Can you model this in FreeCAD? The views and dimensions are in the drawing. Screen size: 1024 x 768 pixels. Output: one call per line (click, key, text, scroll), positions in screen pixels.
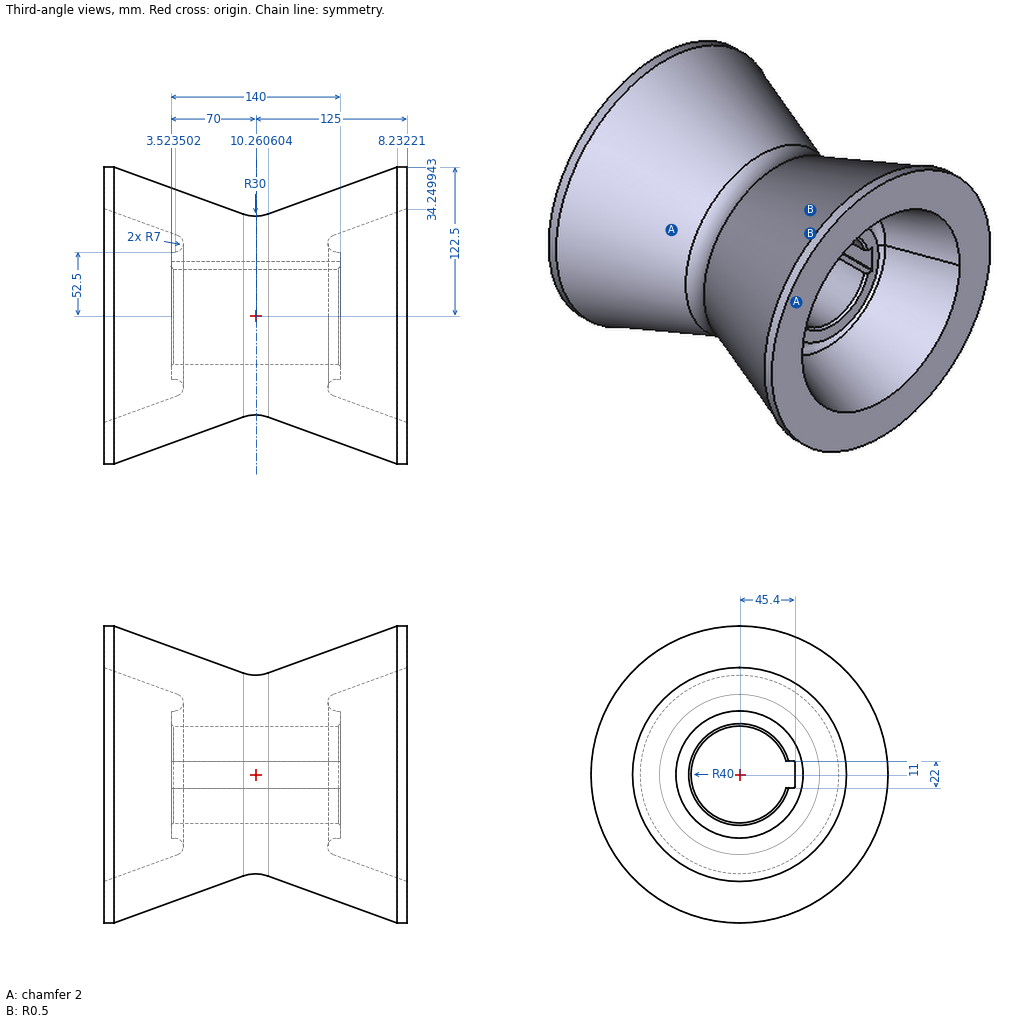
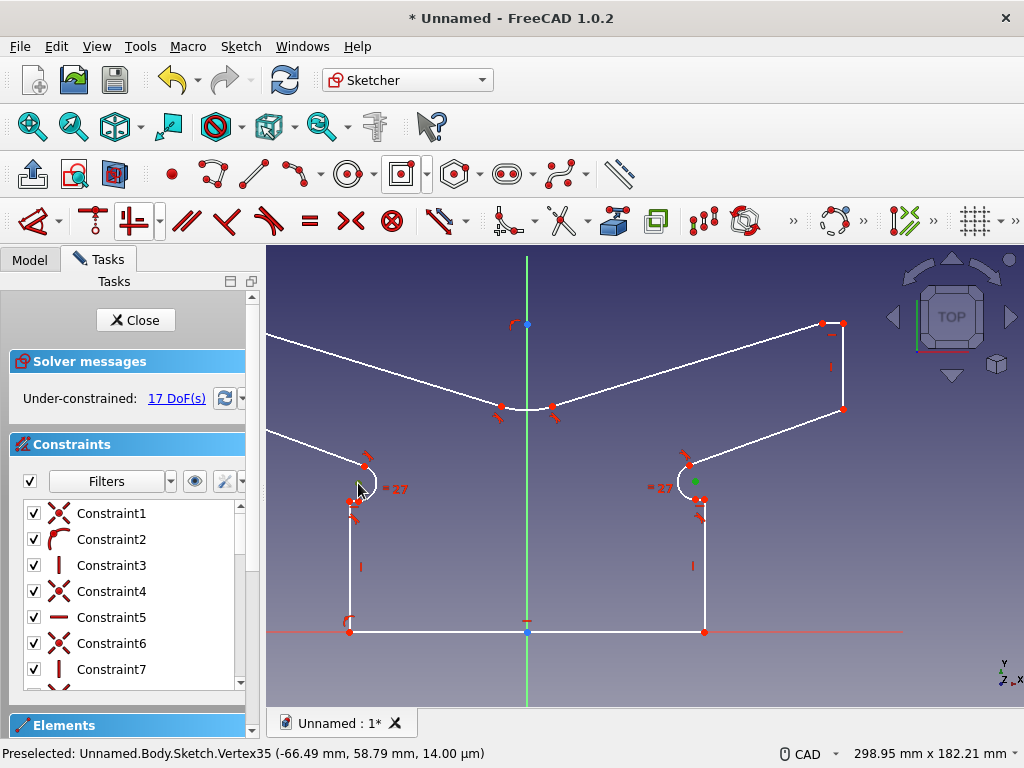
click(527, 592)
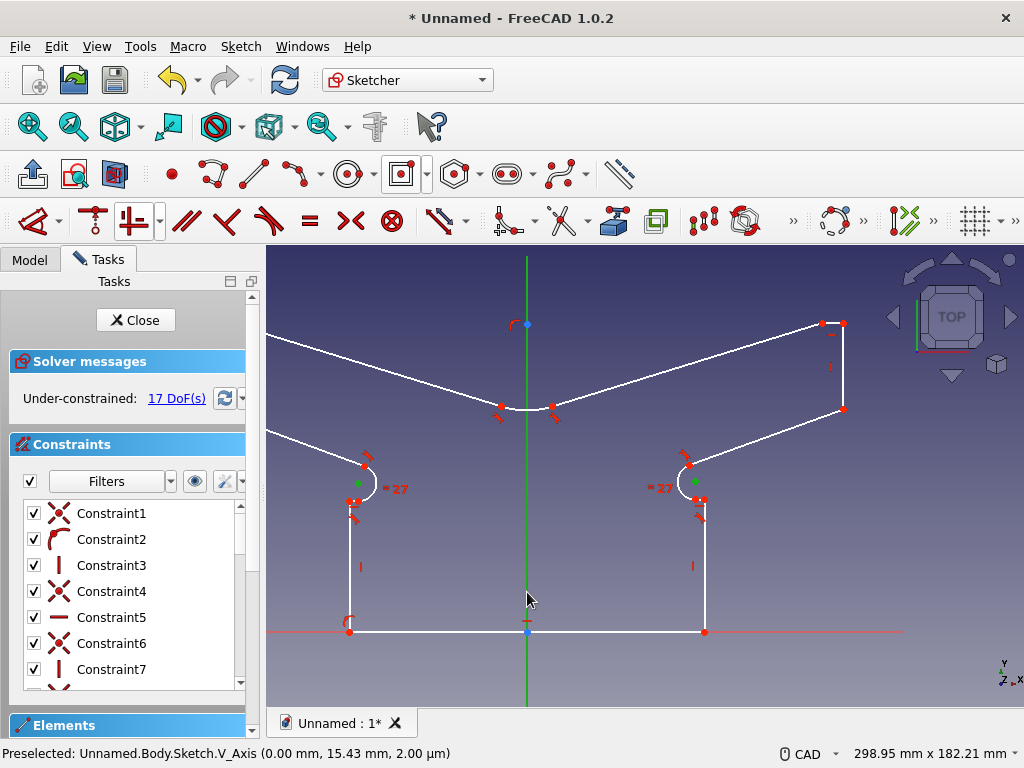
key(s)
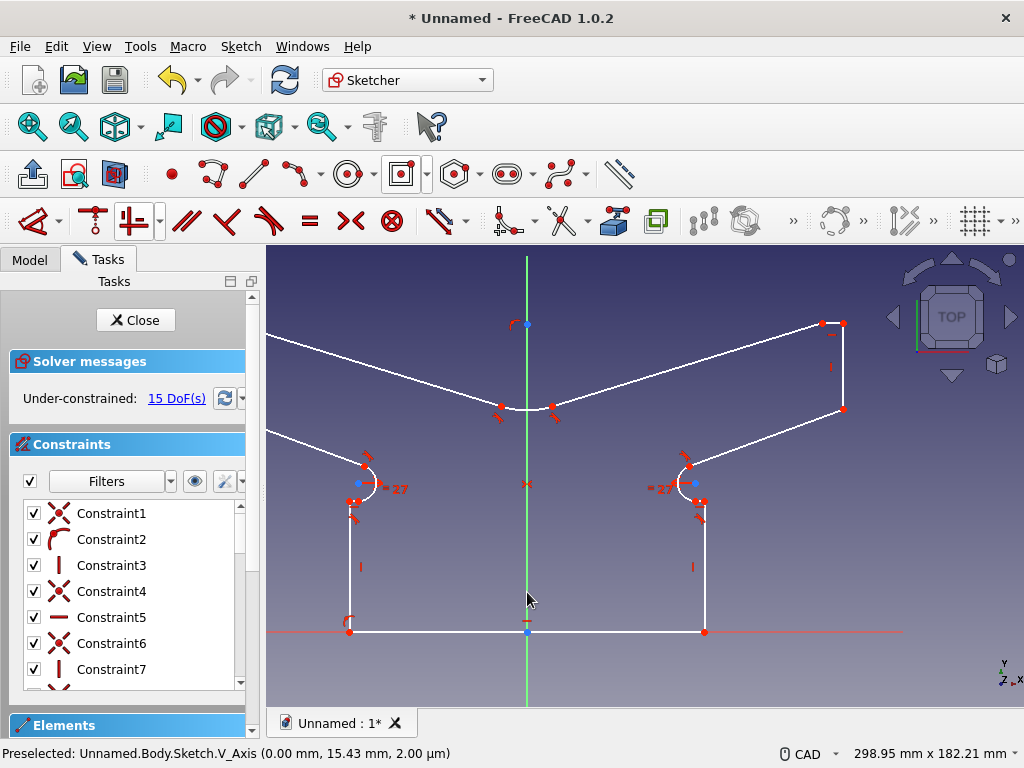
click(822, 323)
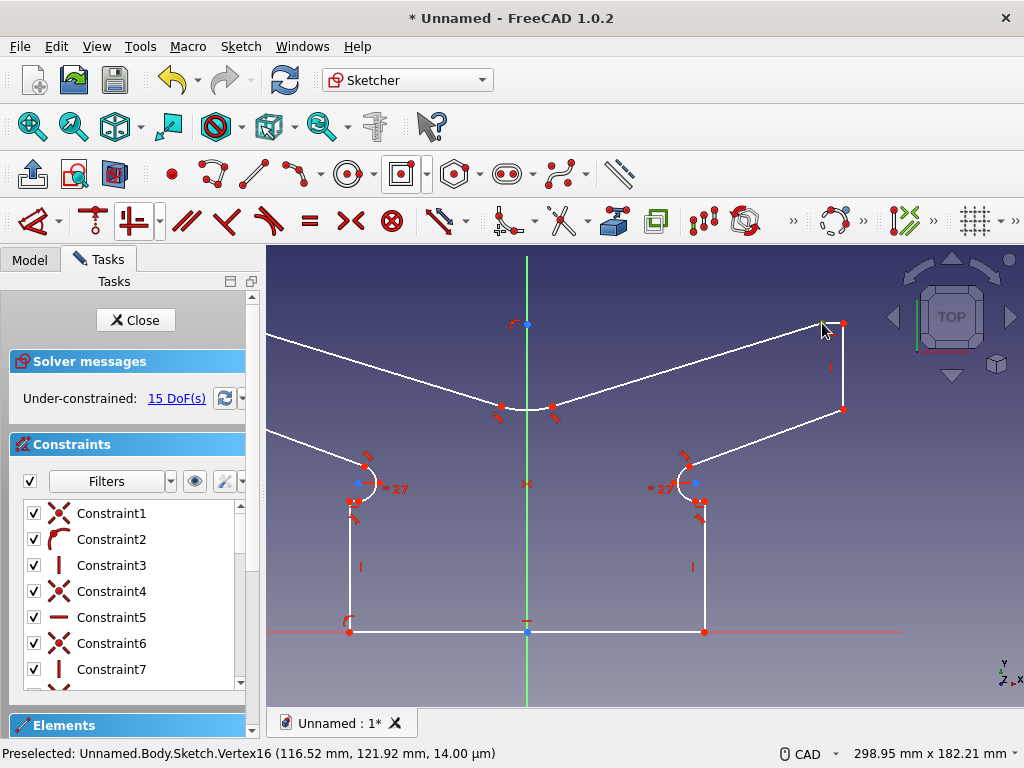
scroll(677, 474, down, 2)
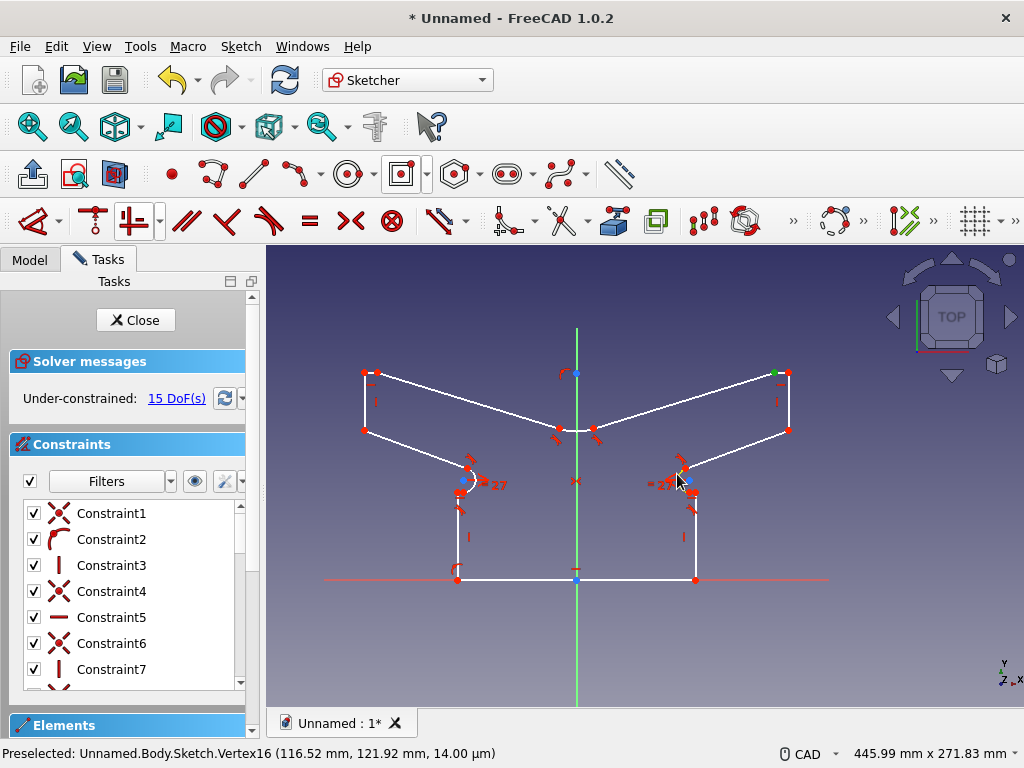
click(378, 373)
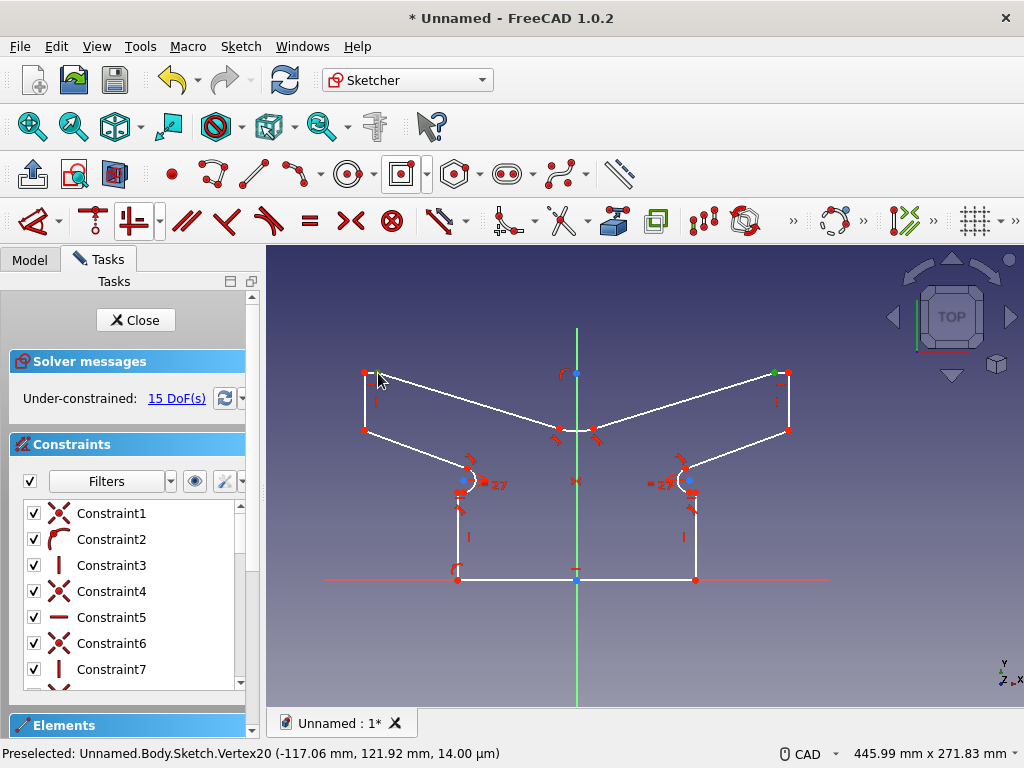
click(577, 650)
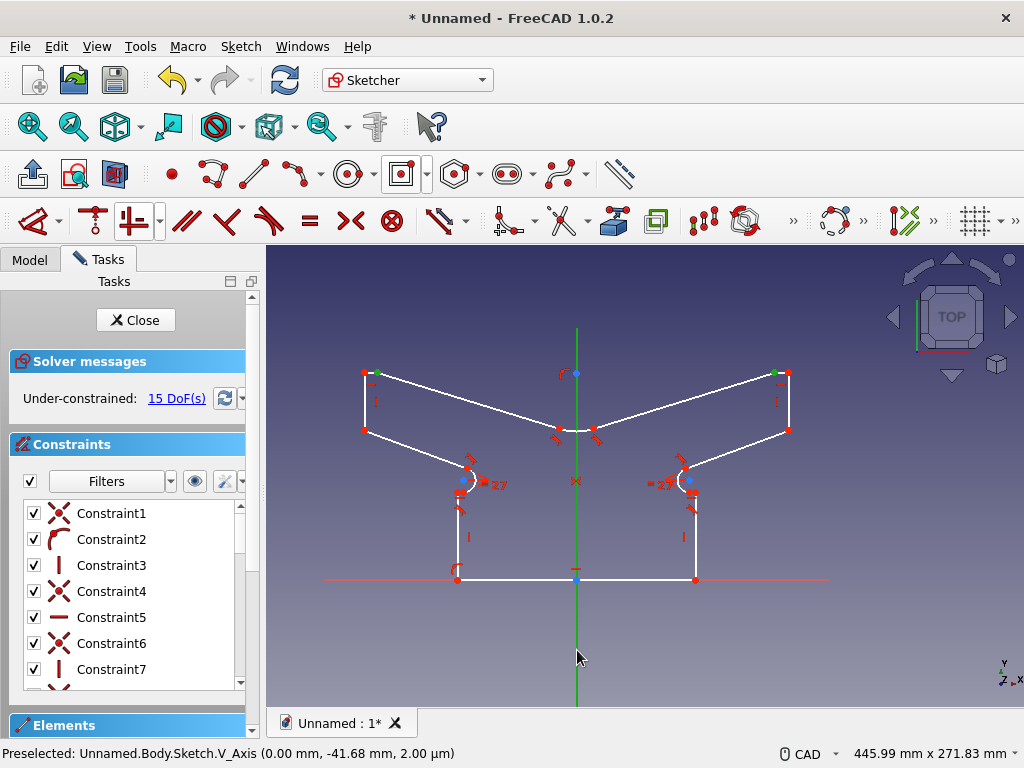
click(351, 222)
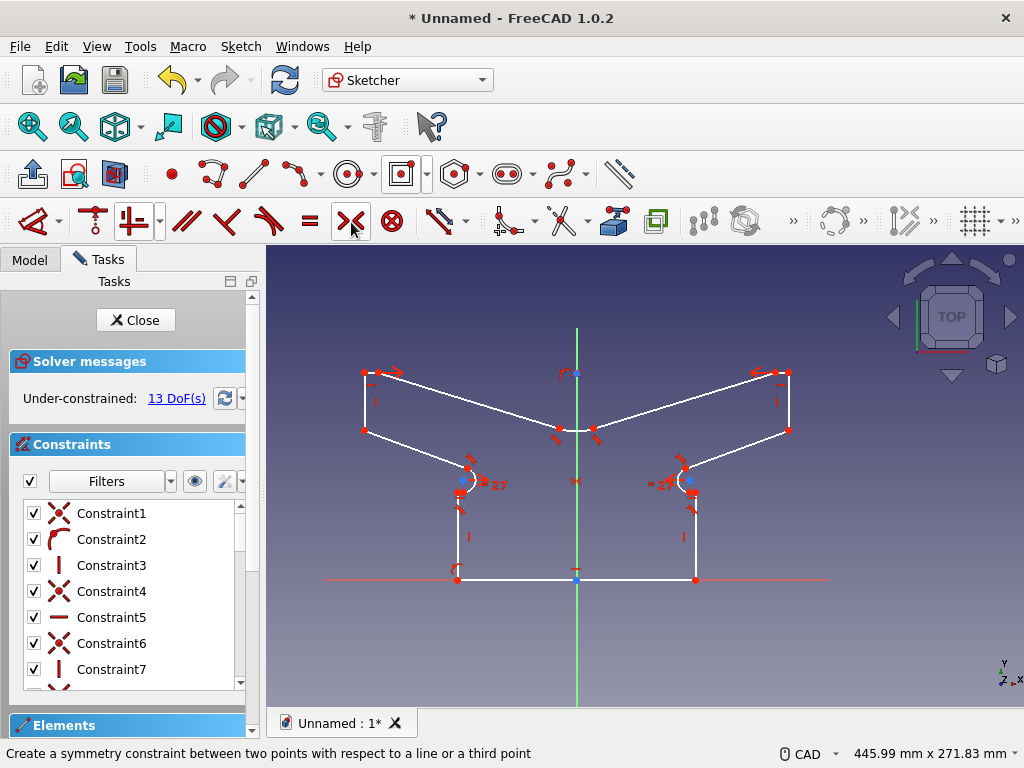
click(789, 431)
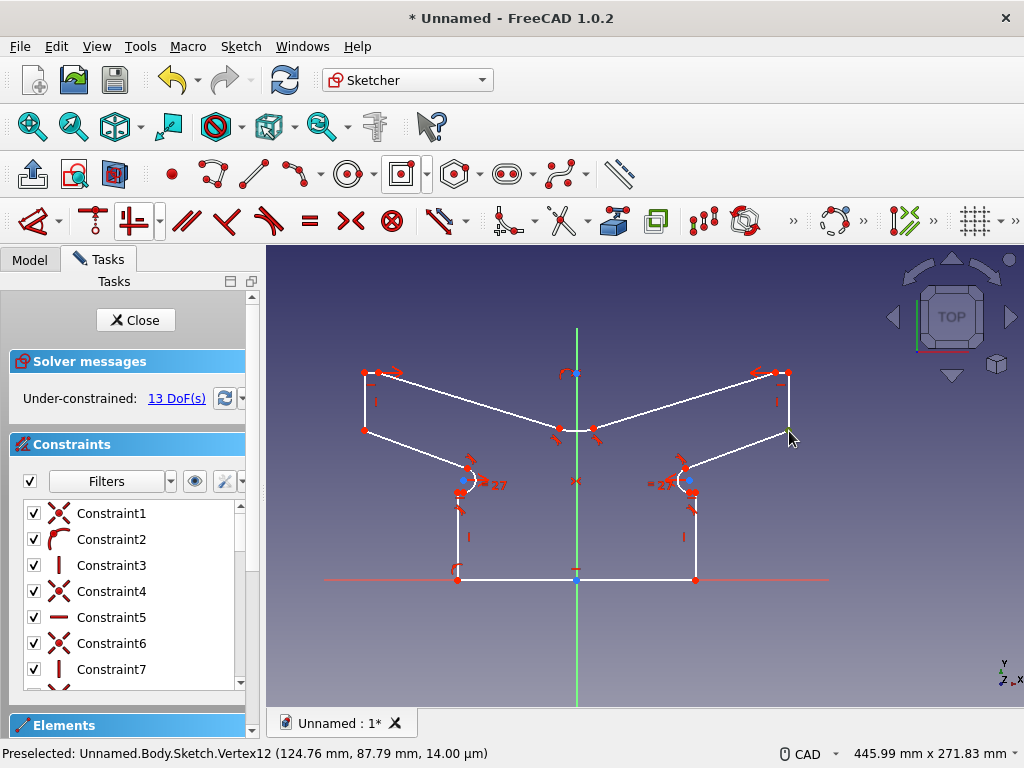
click(365, 431)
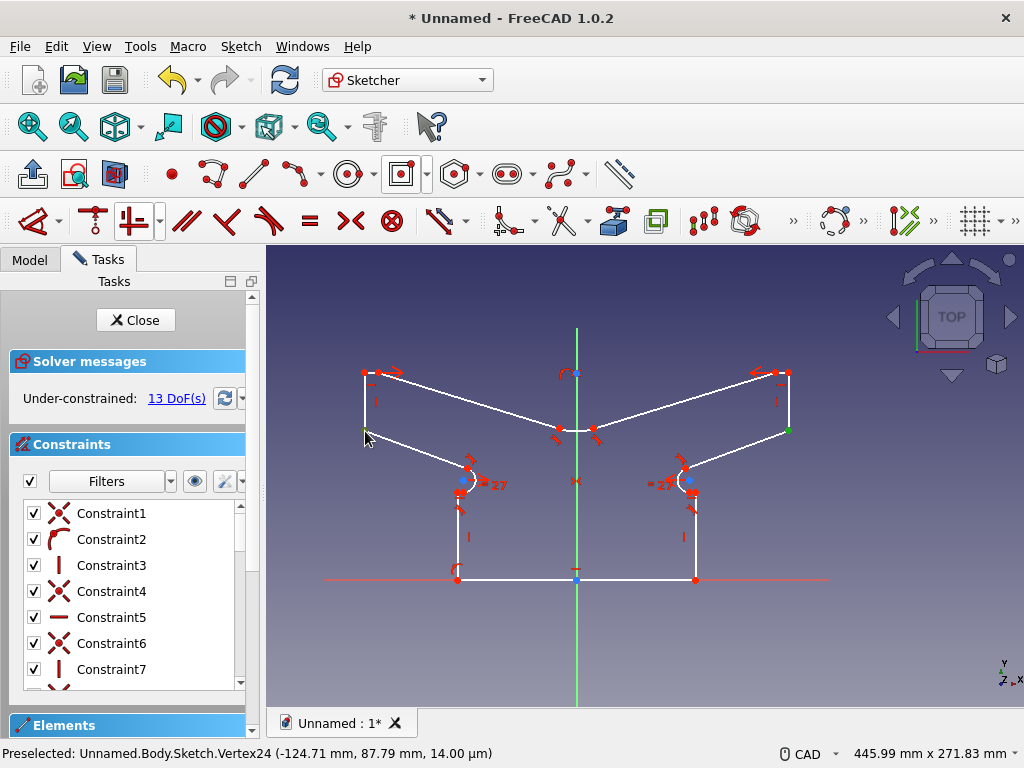
click(577, 650)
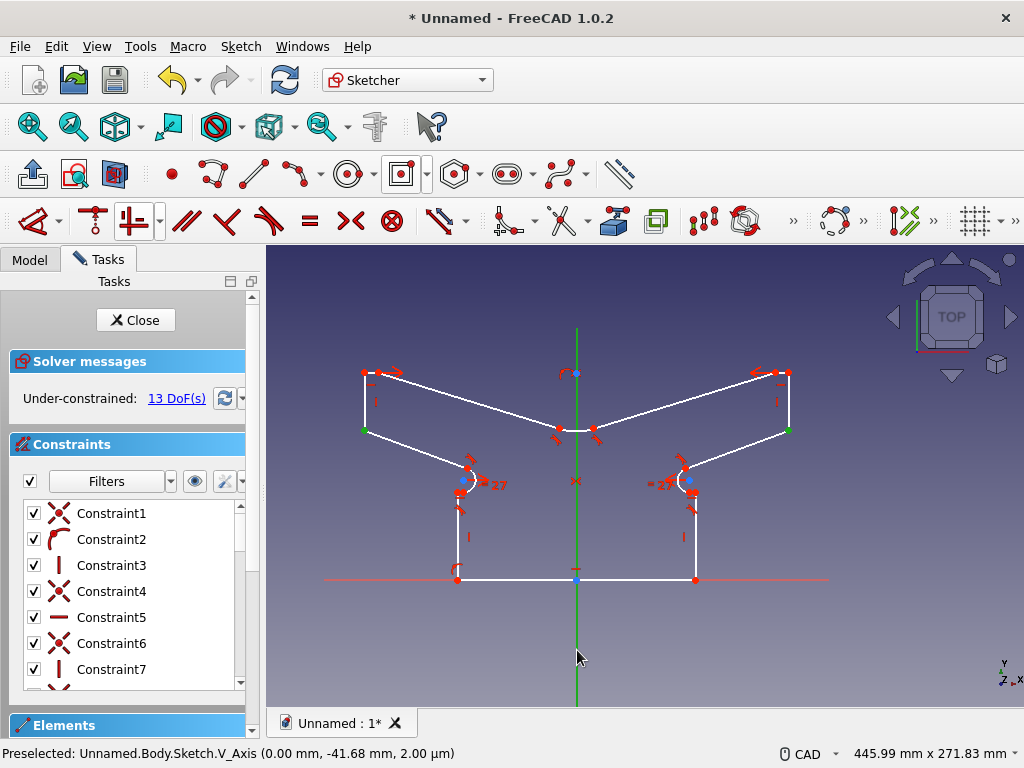
click(351, 222)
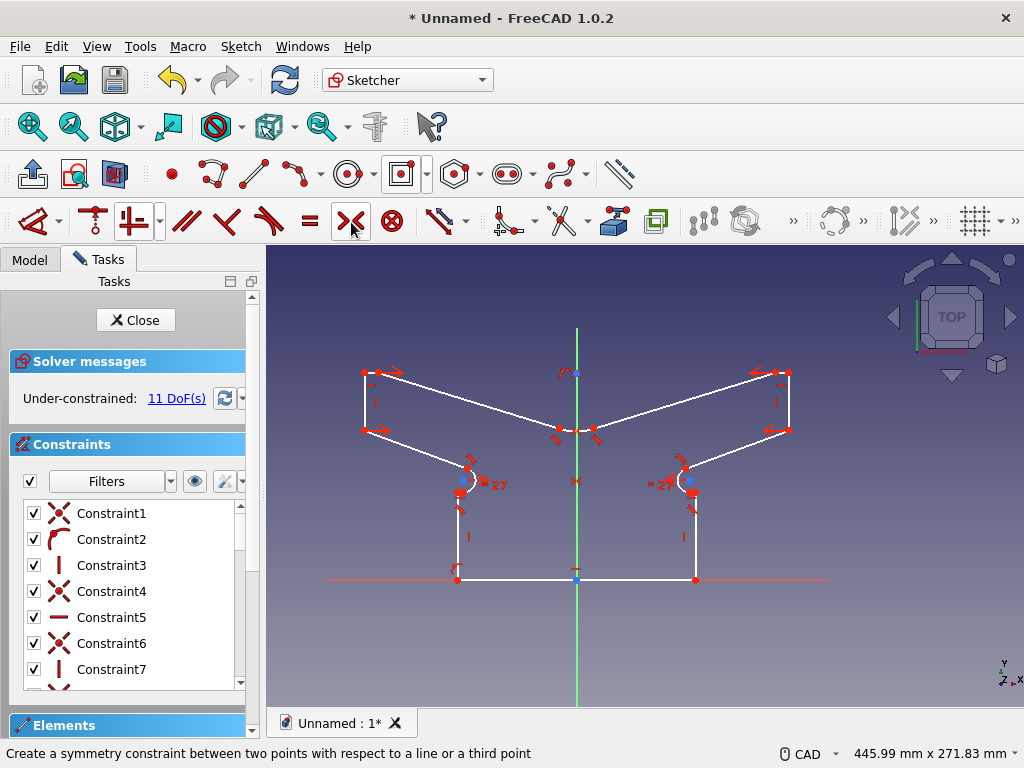
click(32, 222)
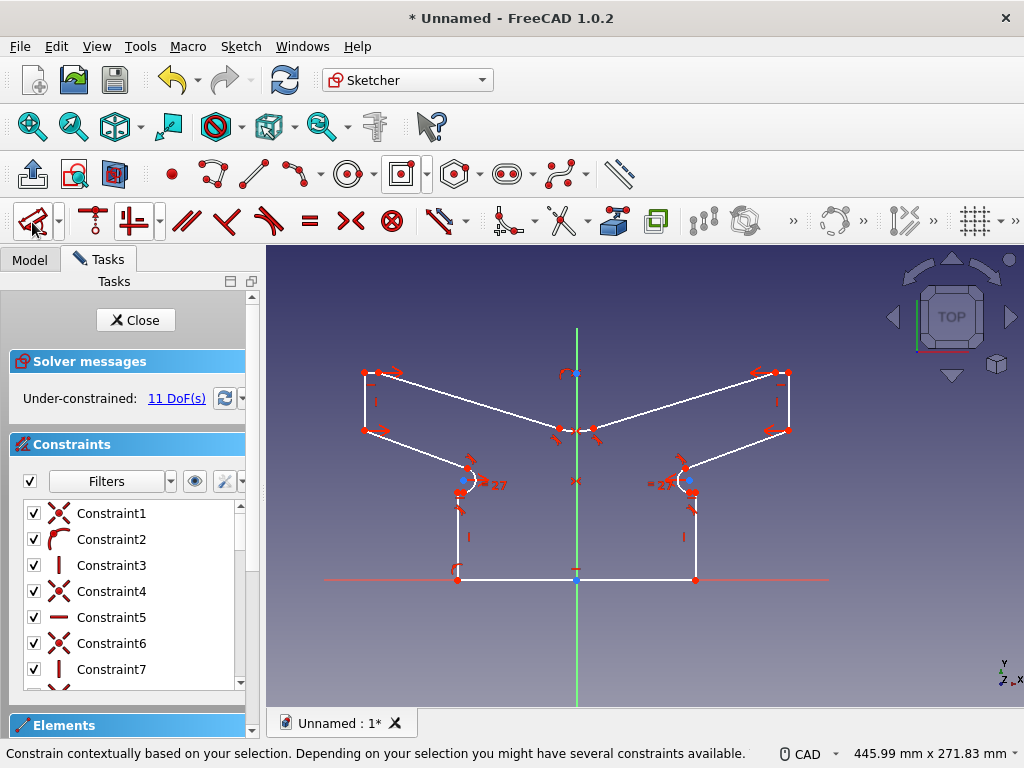
scroll(679, 476, up, 7)